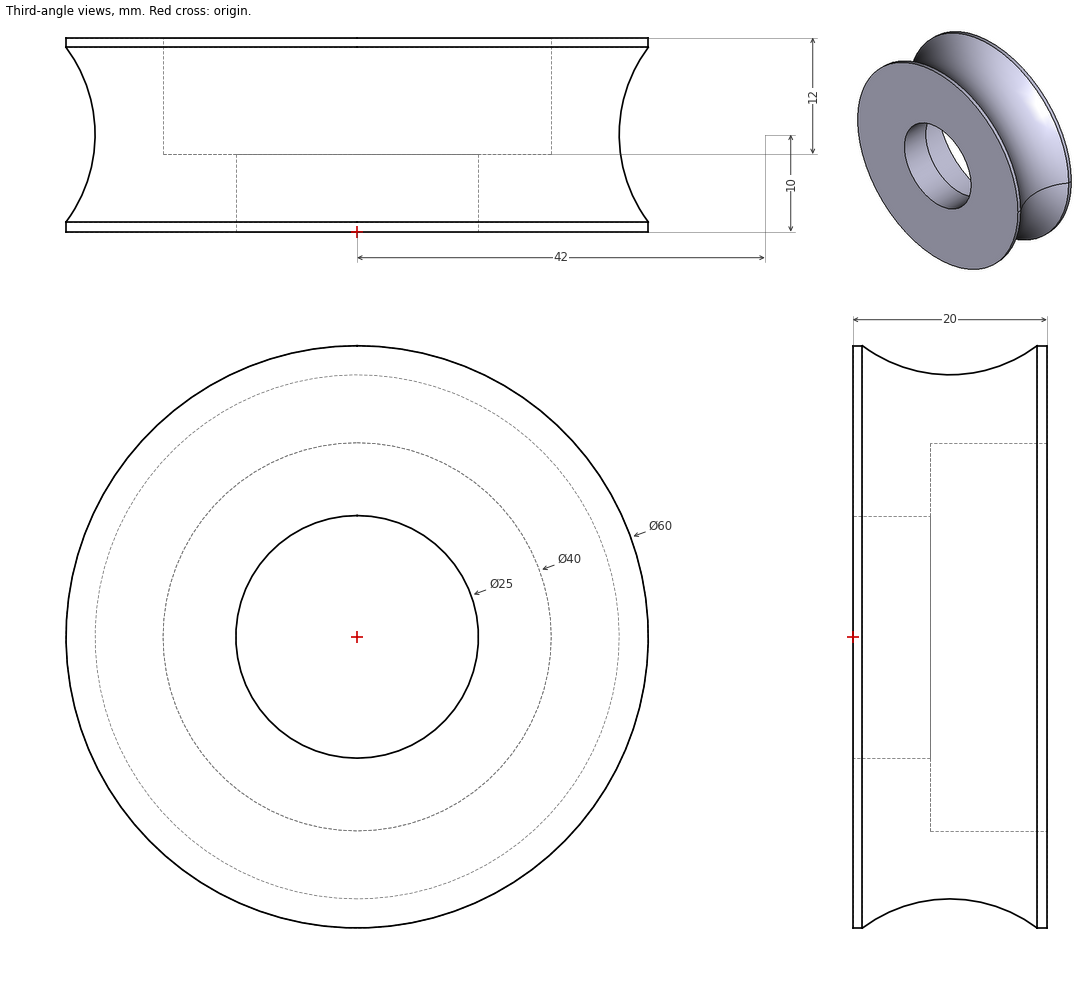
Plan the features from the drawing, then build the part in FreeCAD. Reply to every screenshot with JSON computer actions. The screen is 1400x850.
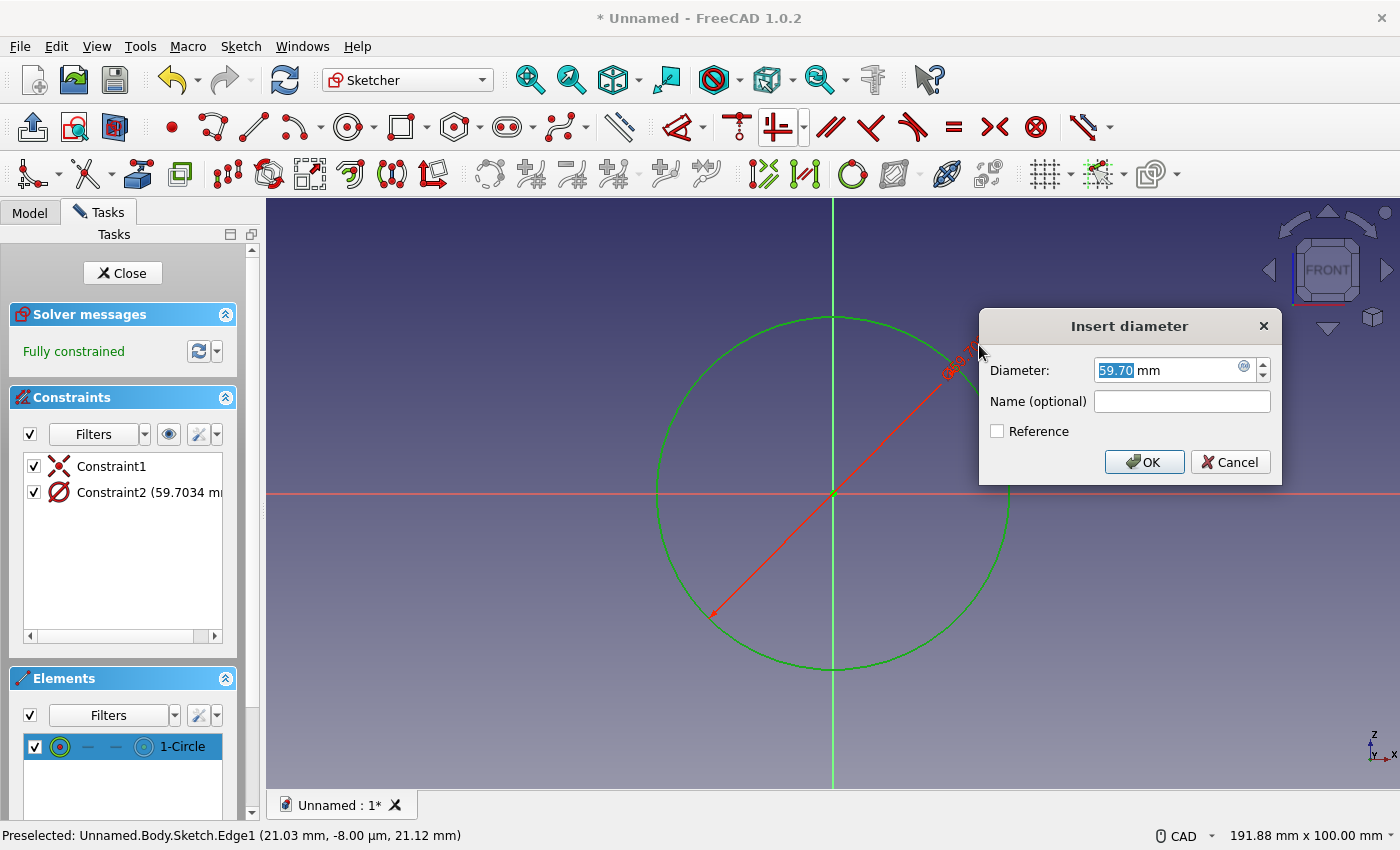
{"action": "type", "text": "60"}
{"action": "key", "text": "Return"}
{"action": "key", "text": "Escape"}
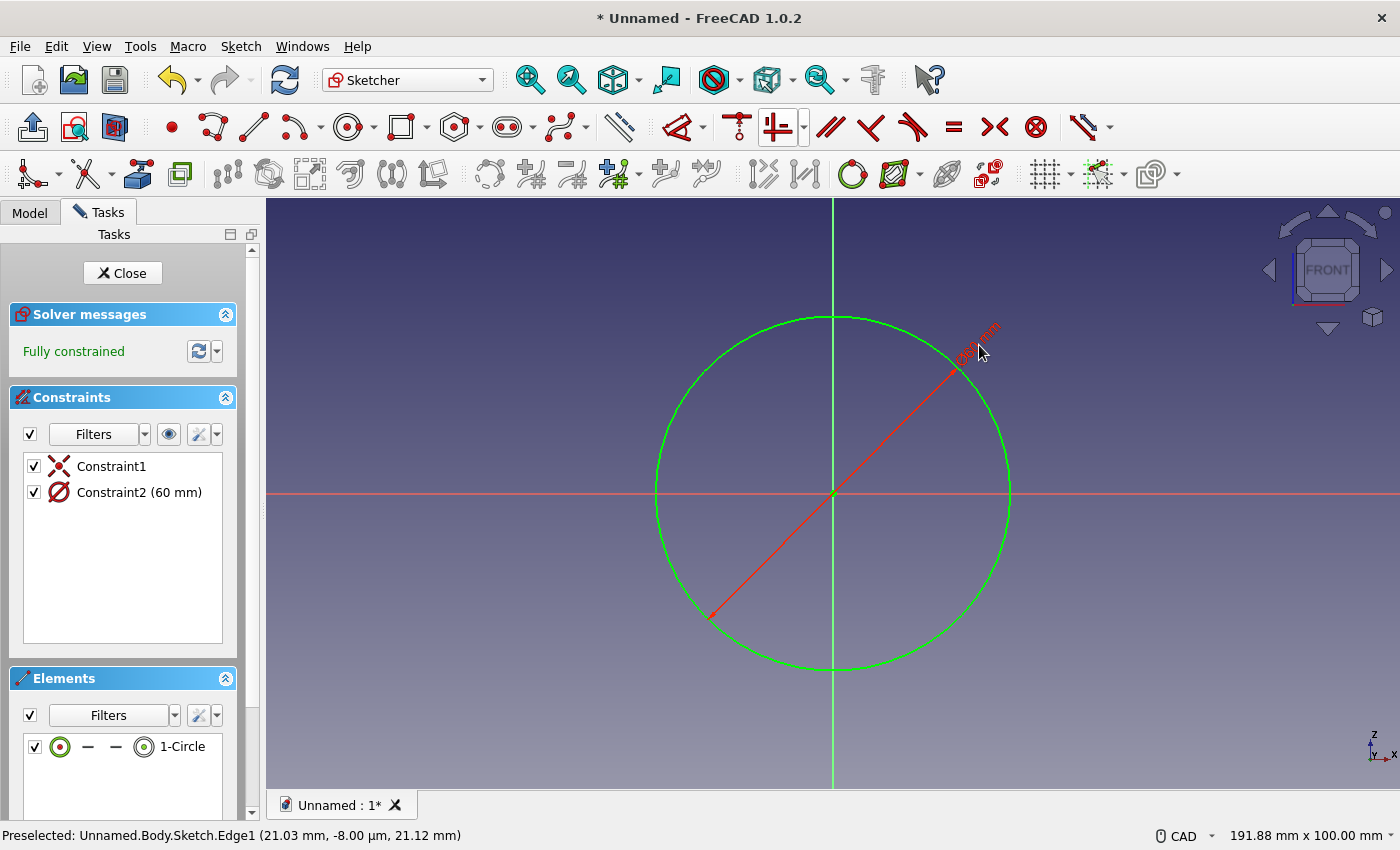
{"action": "left_click", "coordinate": [123, 273]}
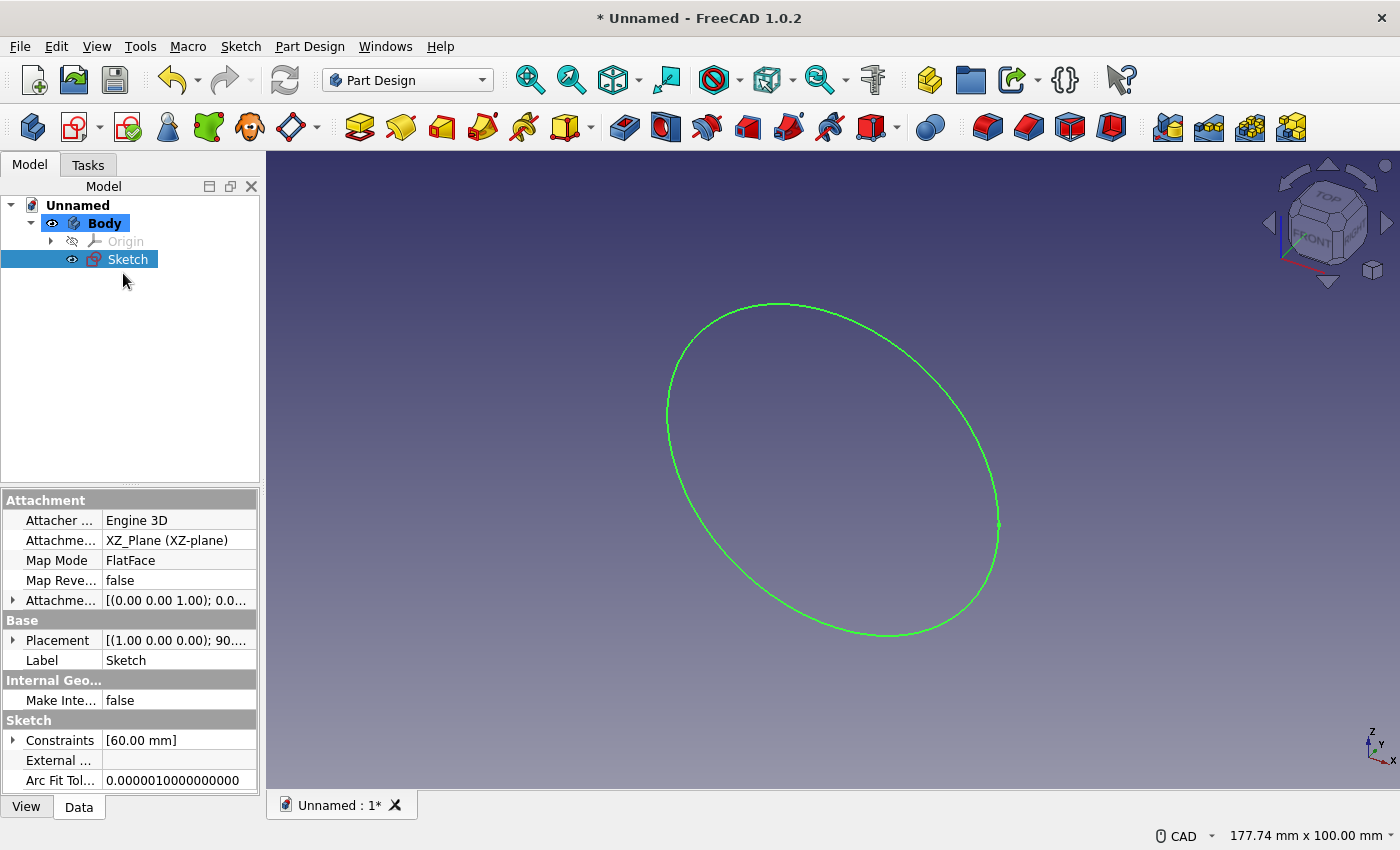
{"action": "left_click", "coordinate": [360, 128]}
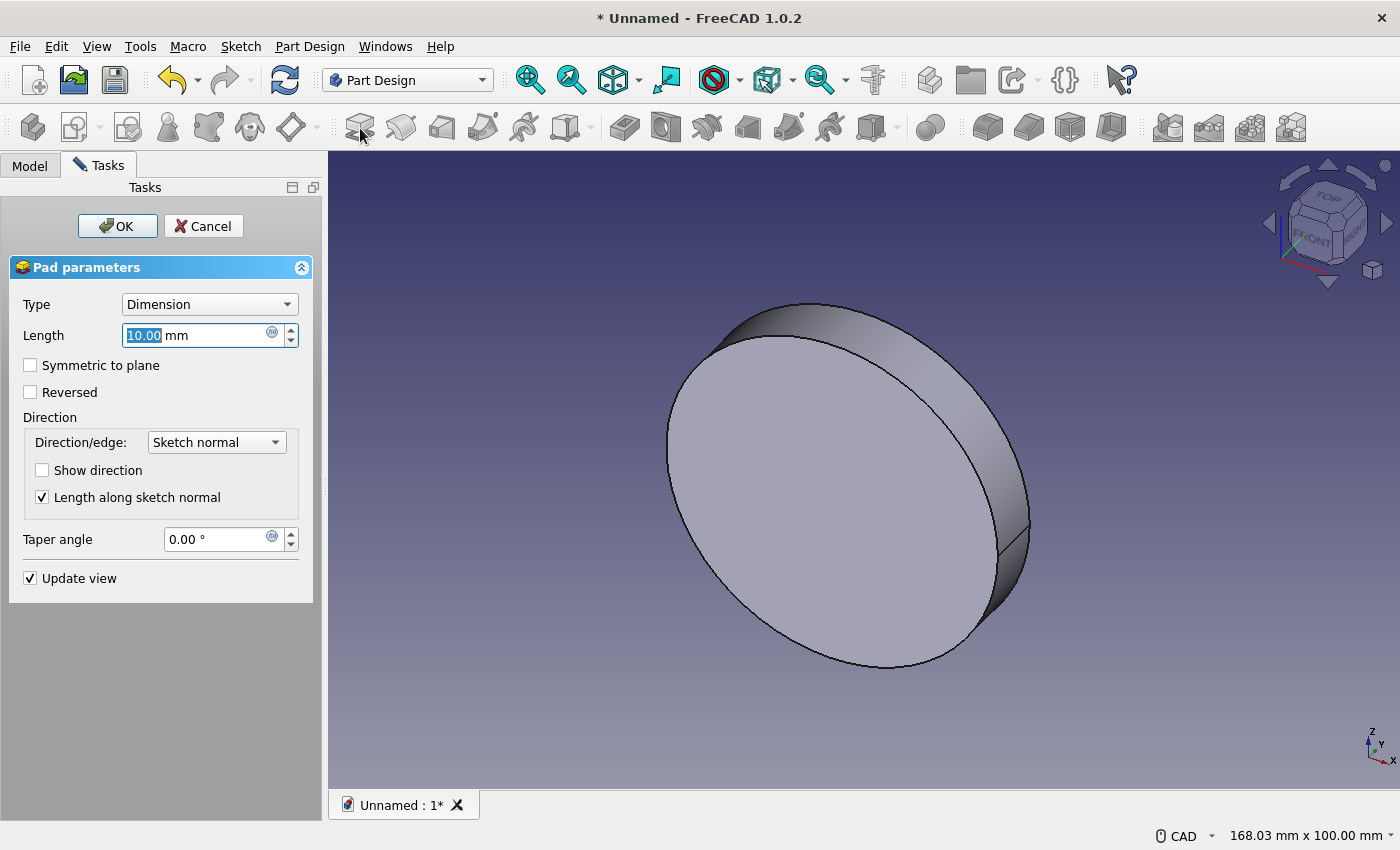
{"action": "type", "text": "20"}
{"action": "key", "text": "Tab"}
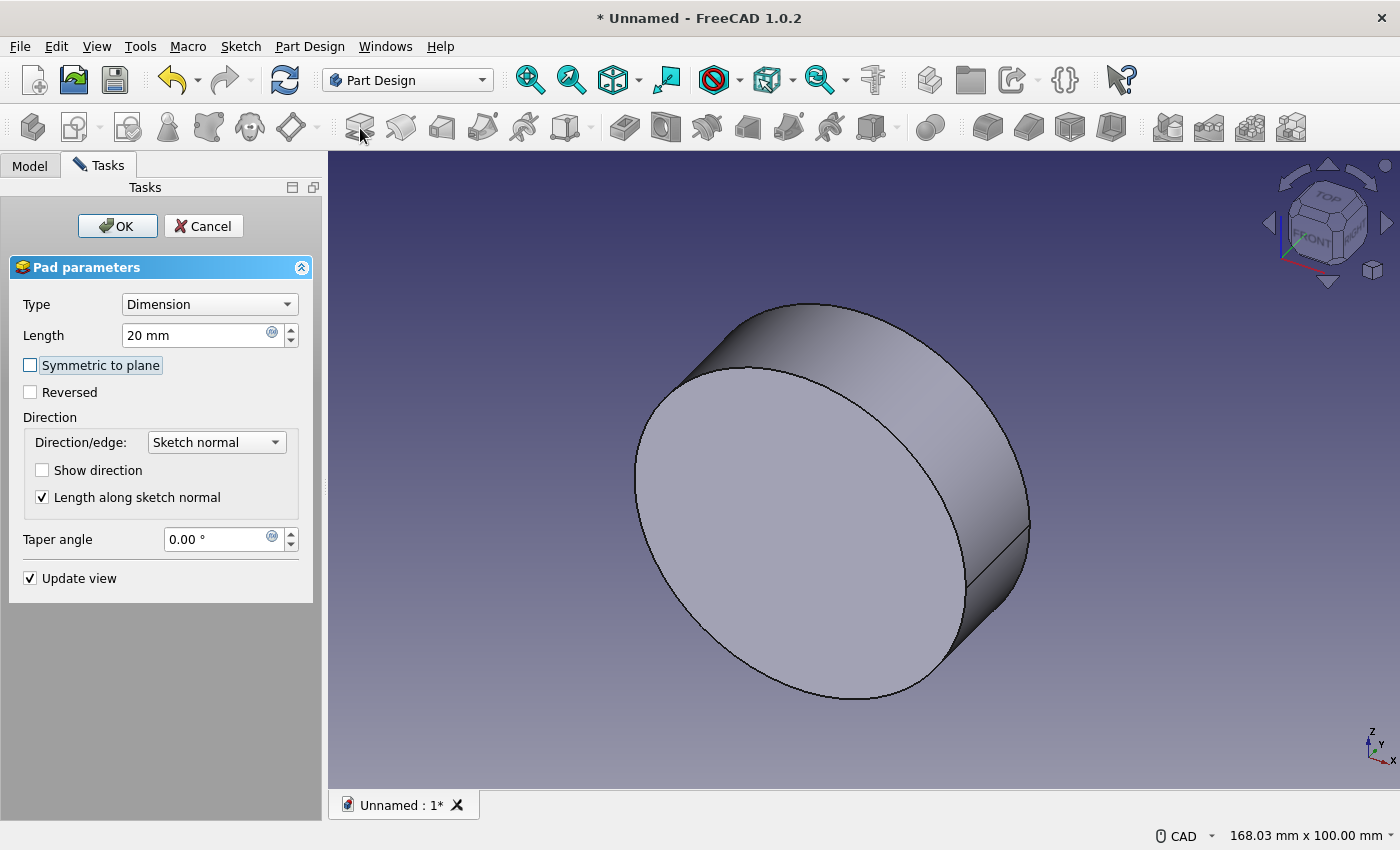
{"action": "left_click", "coordinate": [31, 392]}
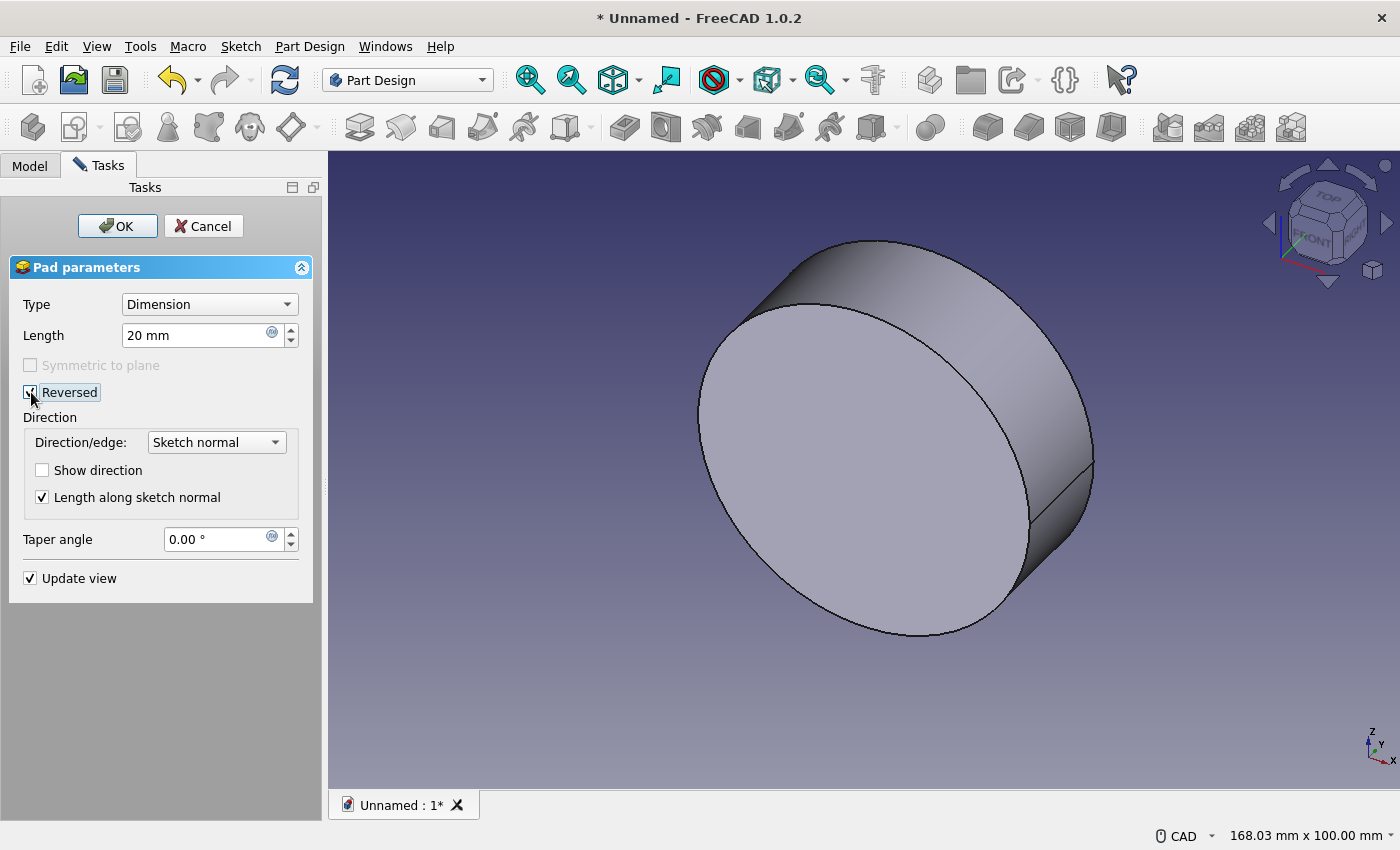
{"action": "left_click", "coordinate": [118, 226]}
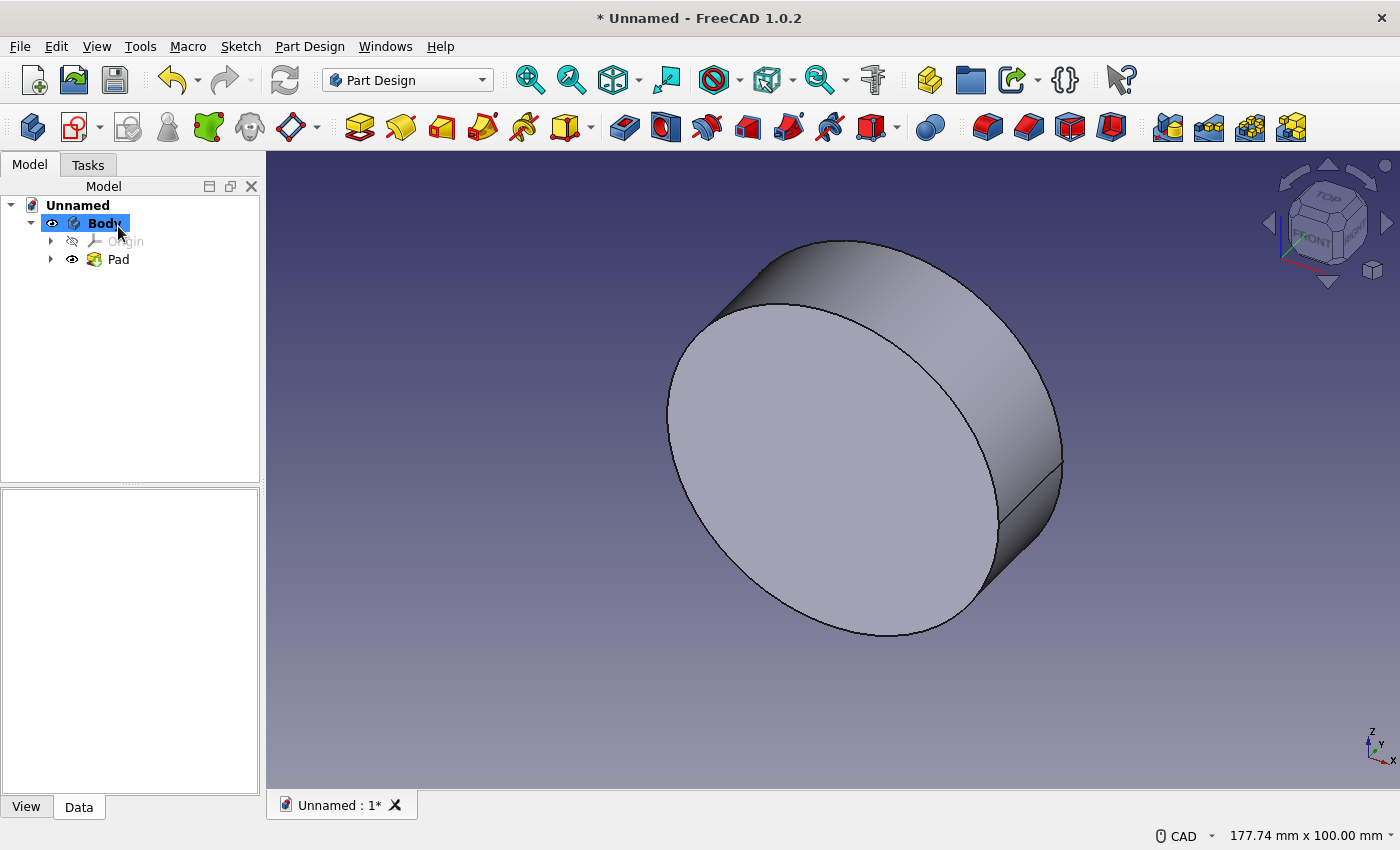
{"action": "key", "text": "4"}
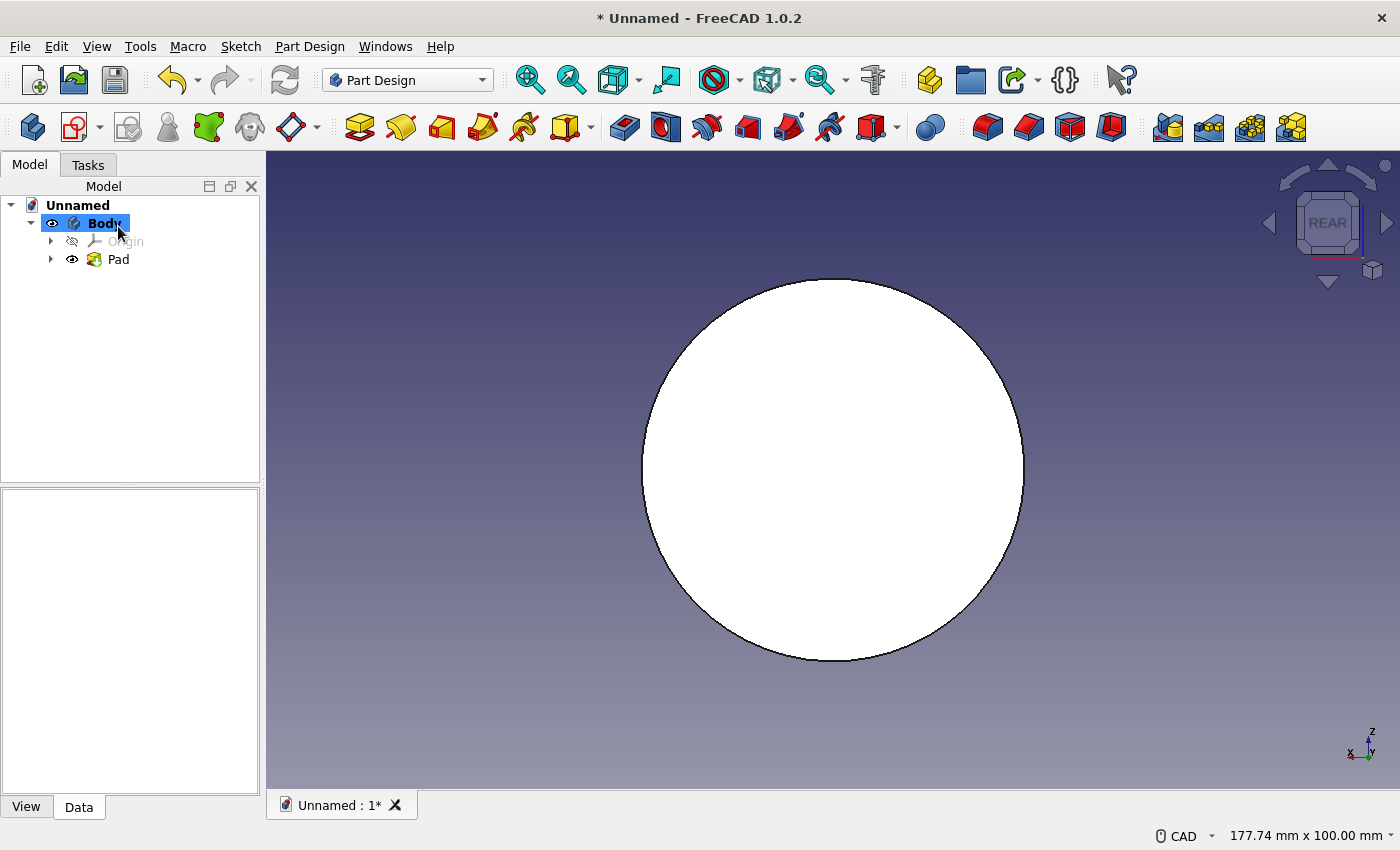
{"action": "left_click", "coordinate": [833, 469]}